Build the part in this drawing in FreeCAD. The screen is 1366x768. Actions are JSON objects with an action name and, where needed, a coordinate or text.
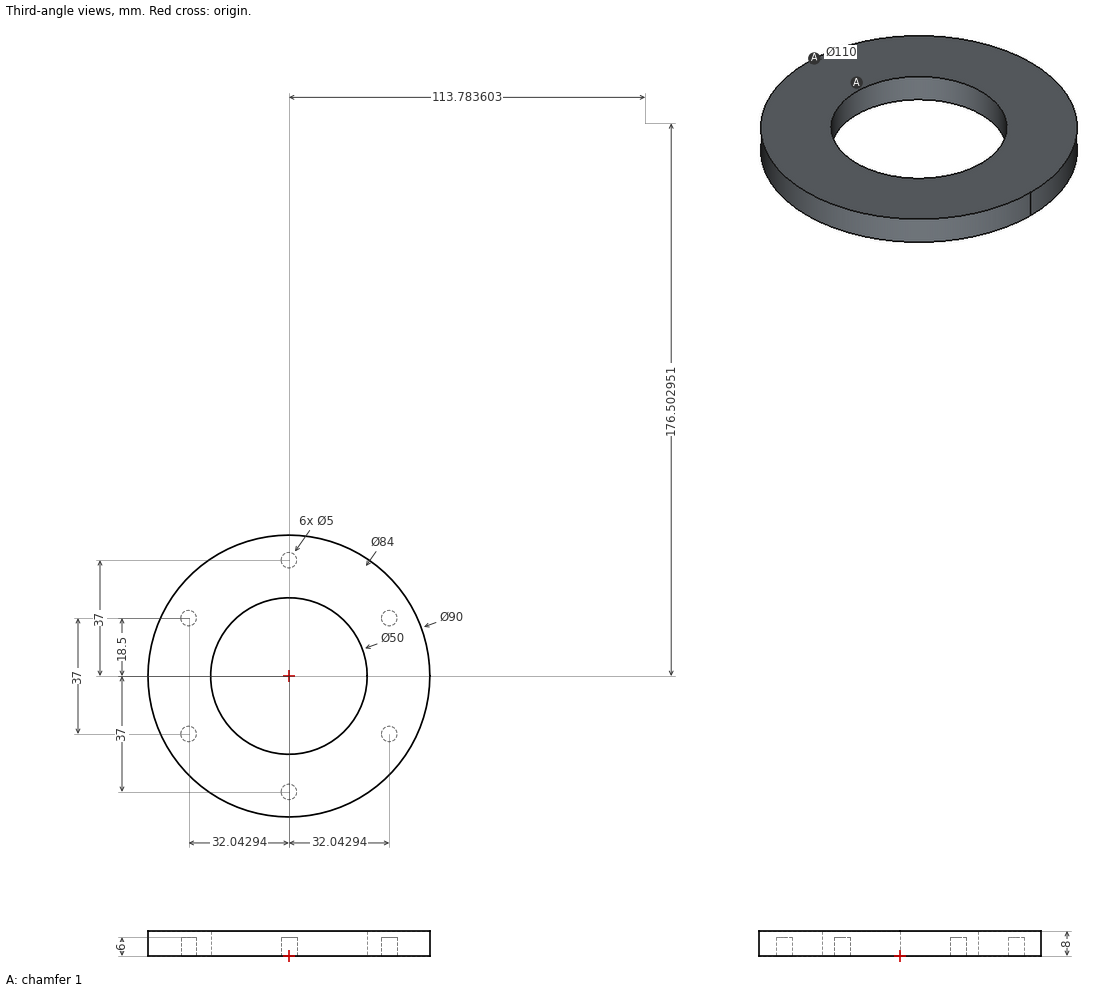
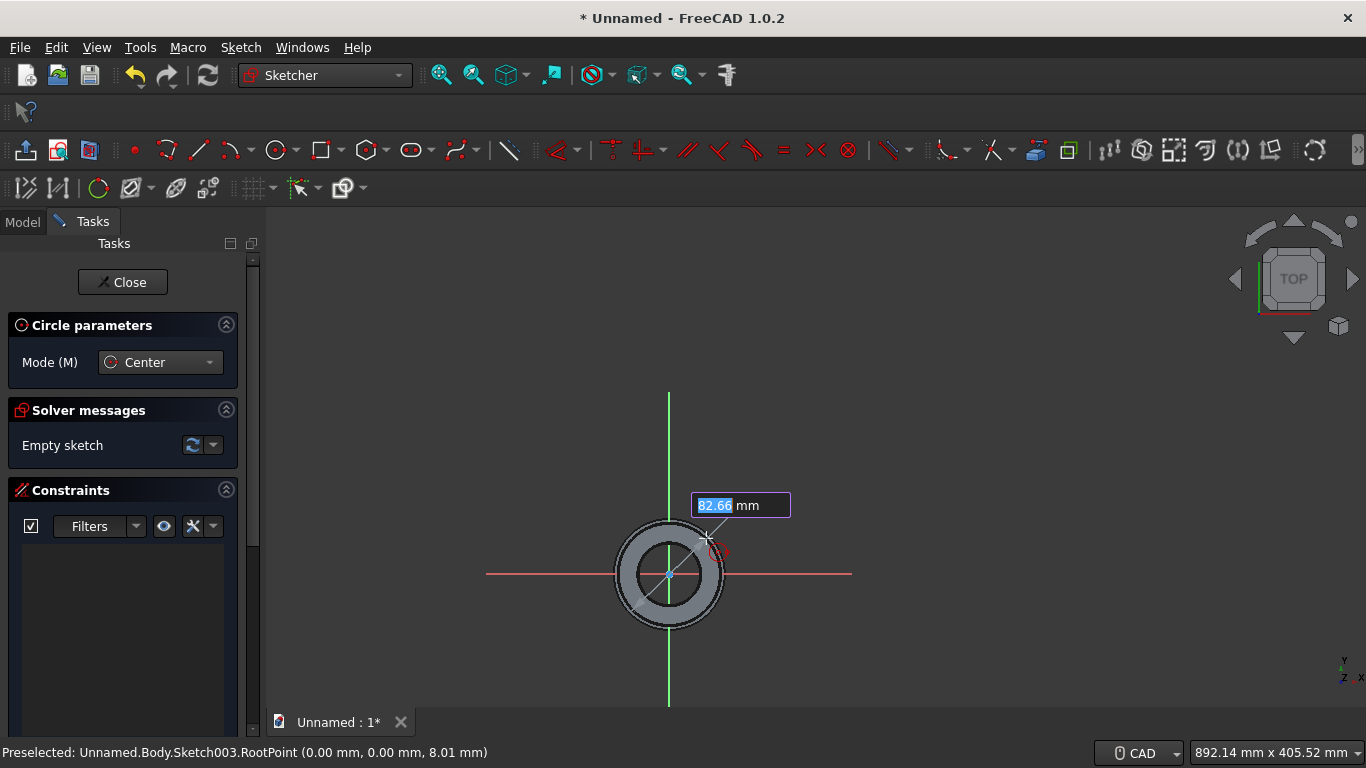
{"action": "type", "text": "84"}
{"action": "key", "text": "Return"}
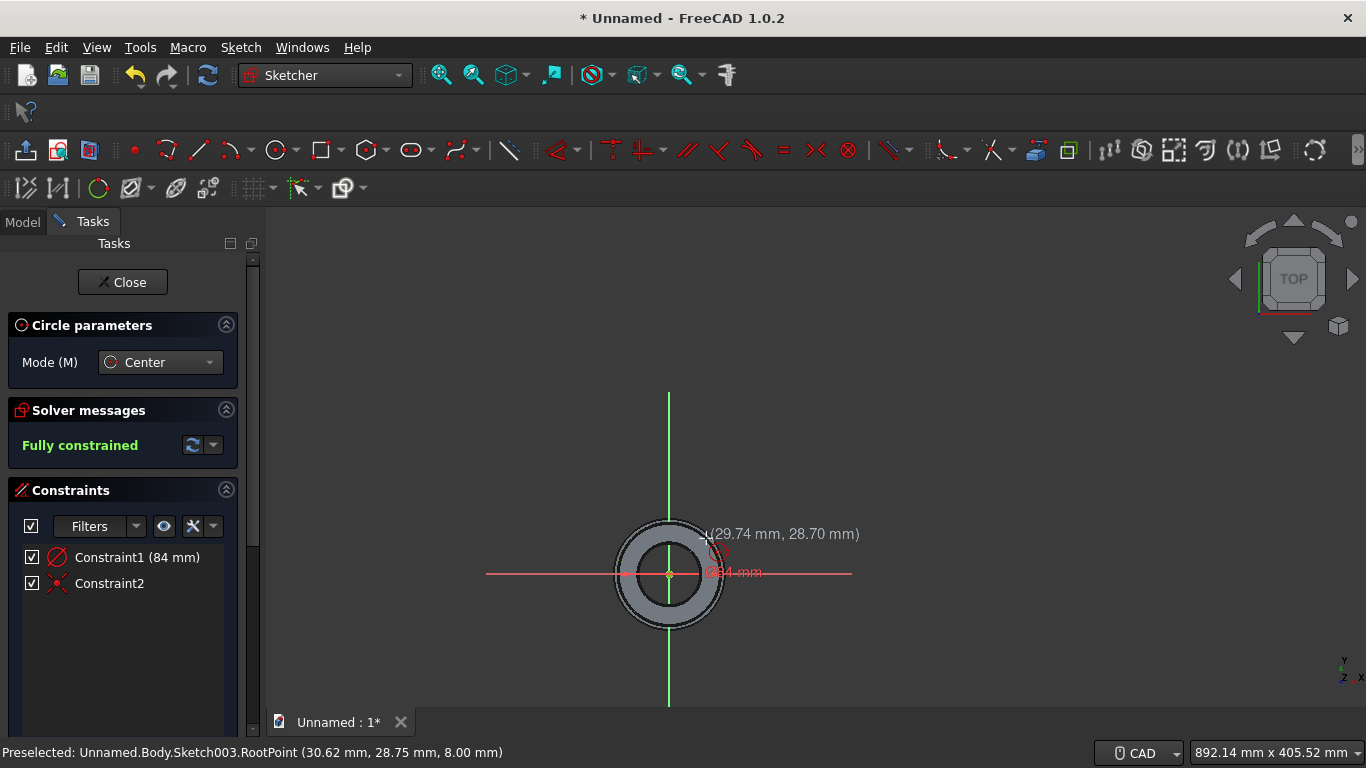
{"action": "left_click", "coordinate": [810, 357]}
{"action": "mouse_move", "coordinate": [858, 309]}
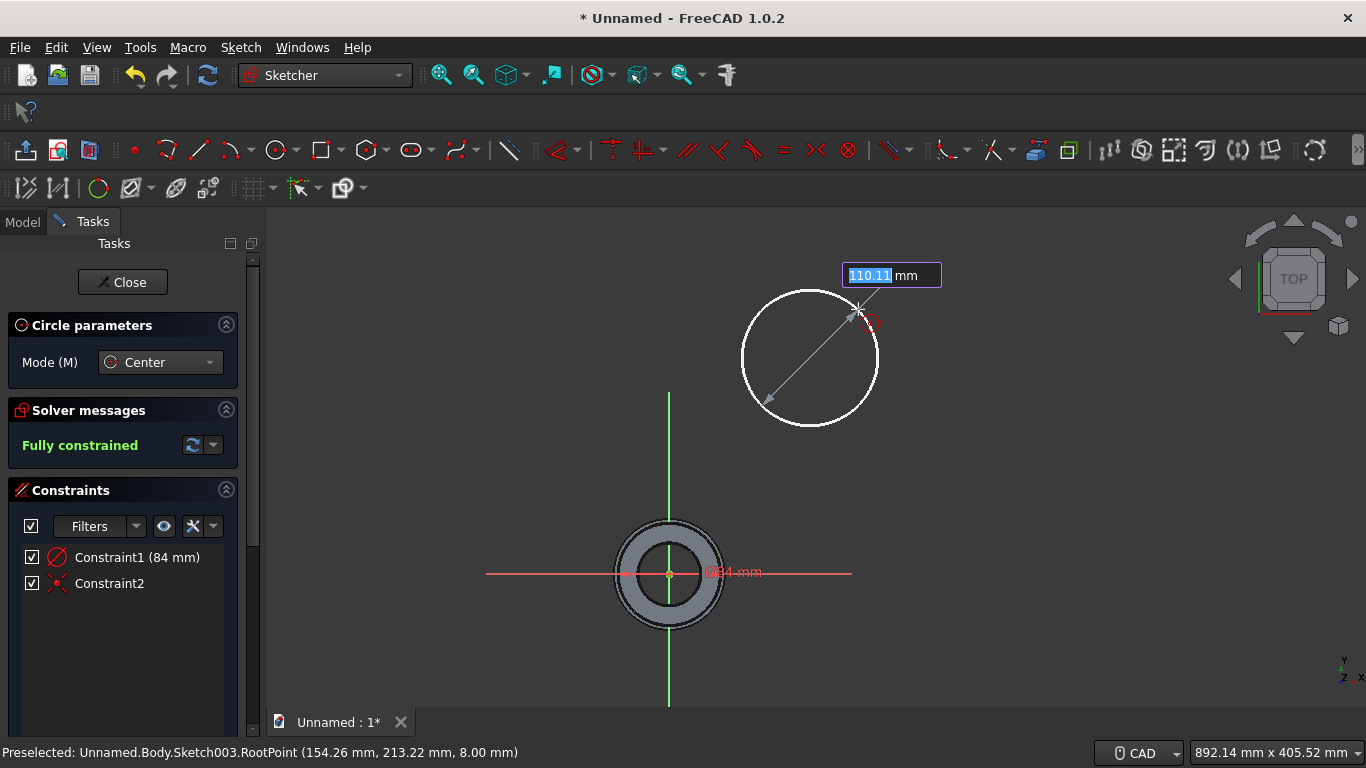
{"action": "type", "text": "110"}
{"action": "key", "text": "Return"}
{"action": "key", "text": "Escape"}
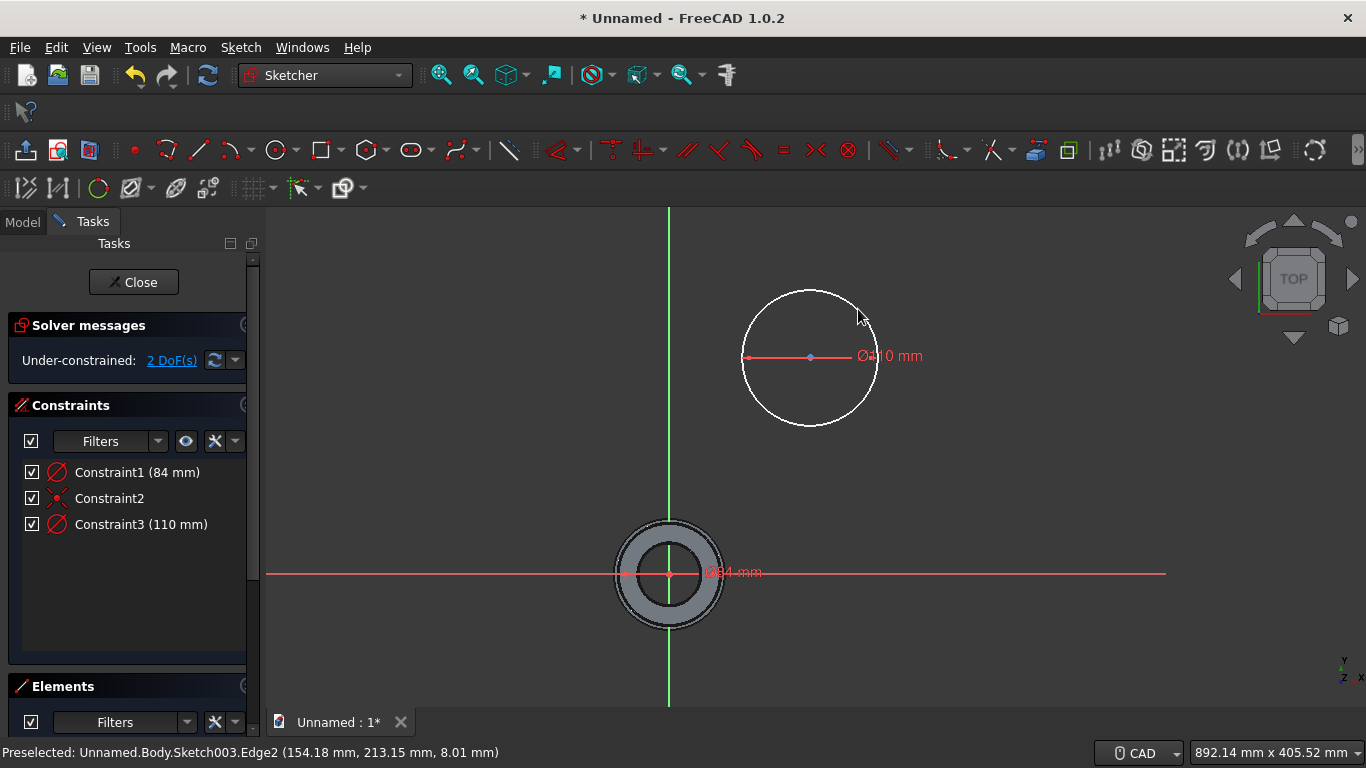
{"action": "key", "text": "d"}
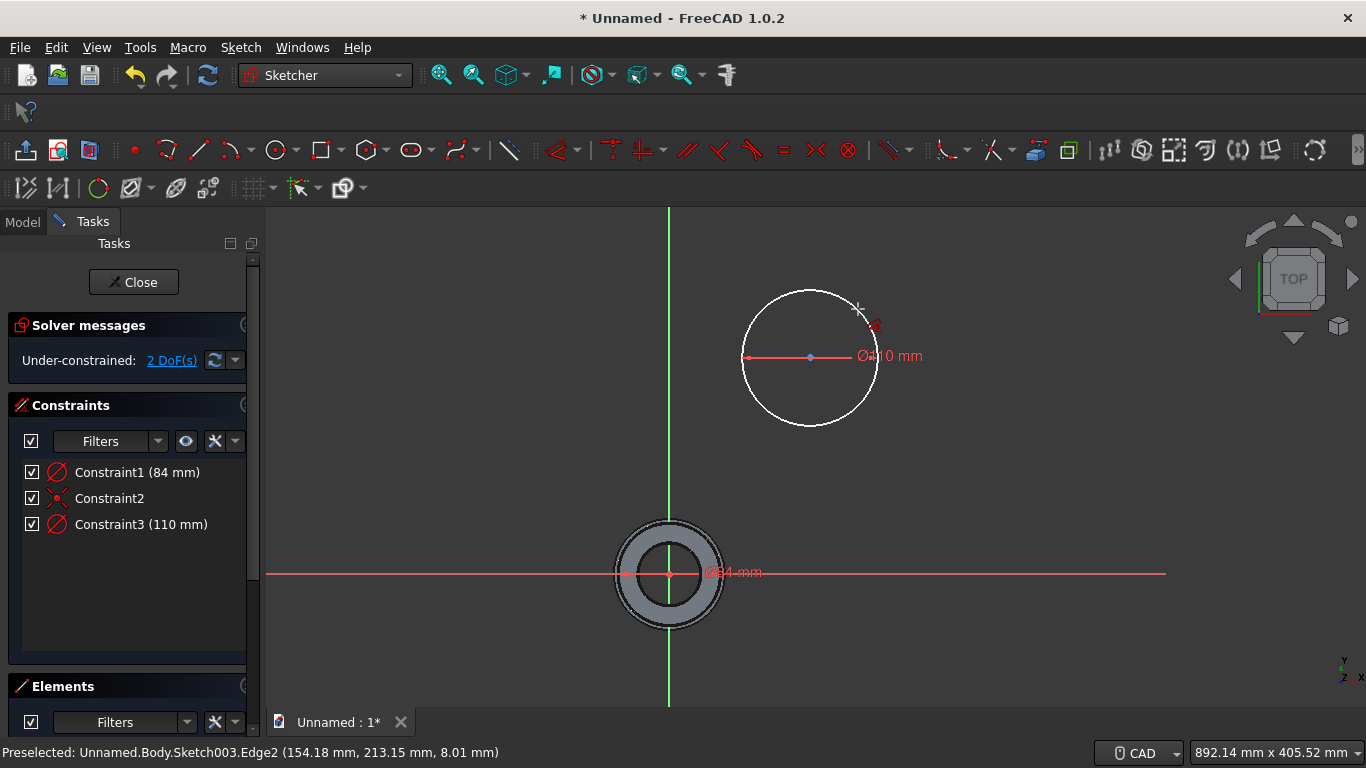
{"action": "left_click", "coordinate": [810, 358]}
{"action": "left_click", "coordinate": [740, 608]}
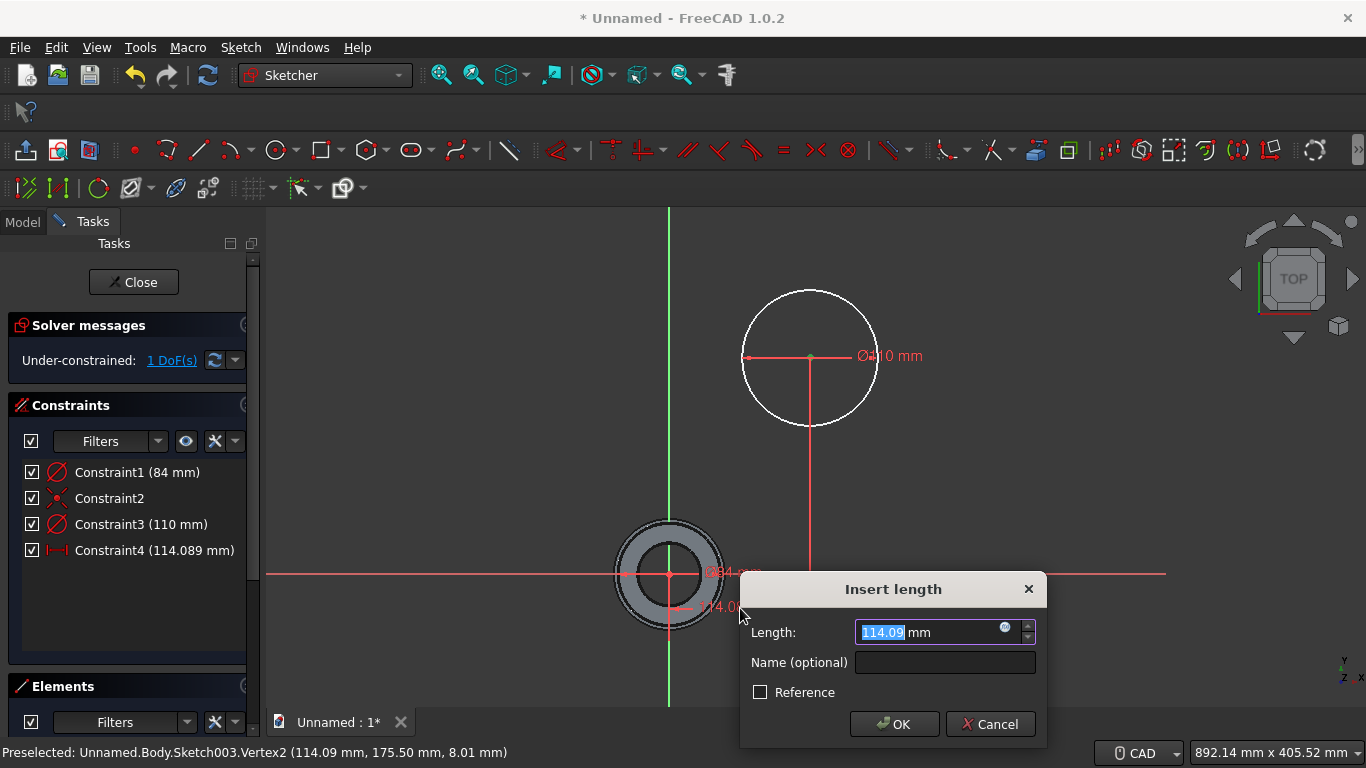
{"action": "type", "text": "113.783603"}
{"action": "key", "text": "Return"}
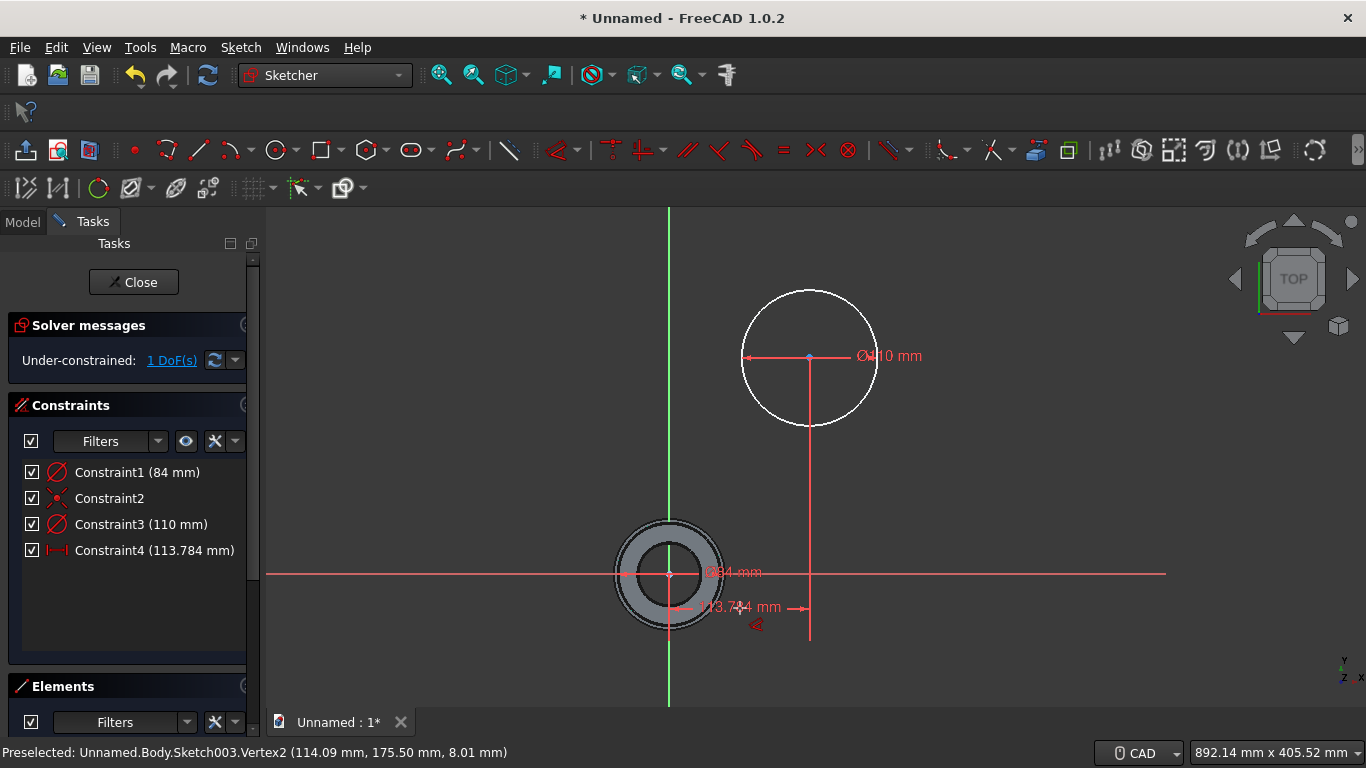
{"action": "left_click", "coordinate": [810, 358]}
{"action": "left_click", "coordinate": [635, 466]}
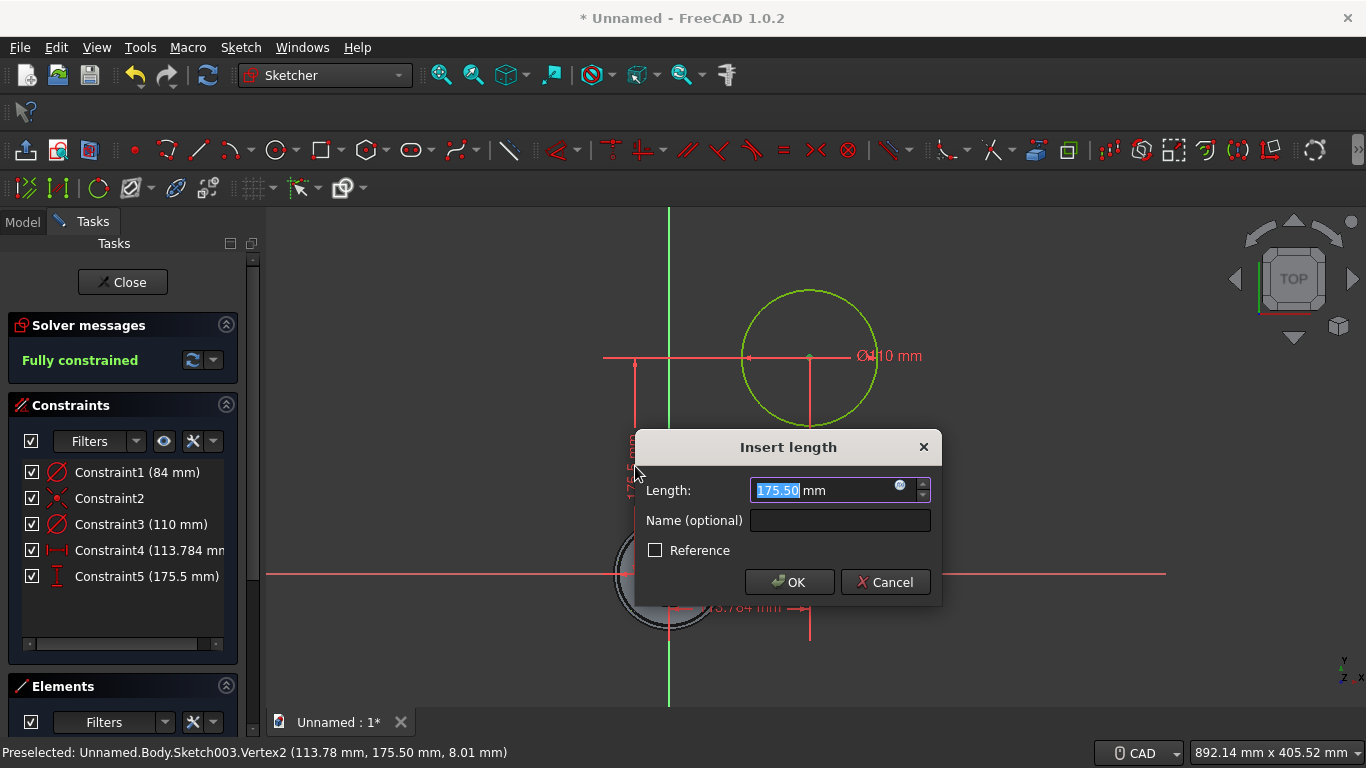
{"action": "type", "text": "176.502951"}
{"action": "key", "text": "Return"}
{"action": "key", "text": "Escape"}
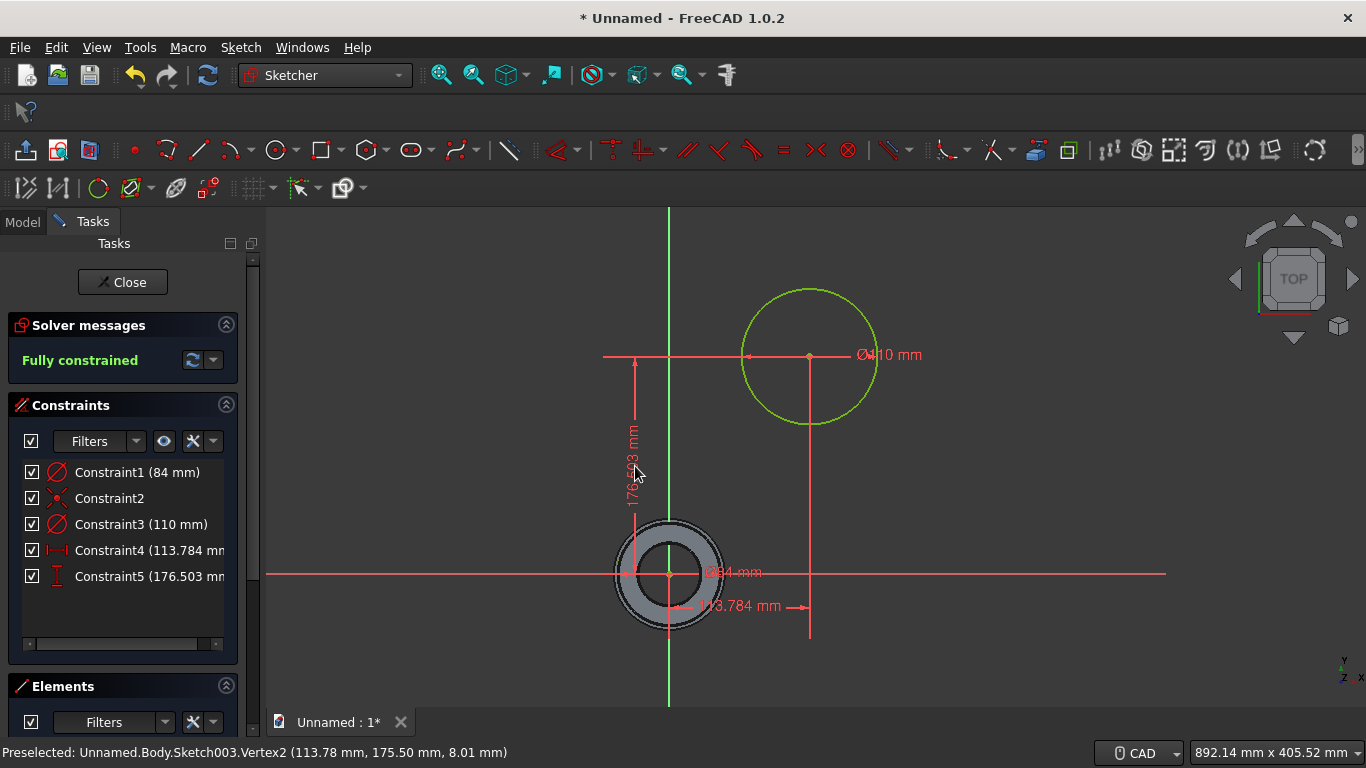
{"action": "left_click", "coordinate": [123, 282]}